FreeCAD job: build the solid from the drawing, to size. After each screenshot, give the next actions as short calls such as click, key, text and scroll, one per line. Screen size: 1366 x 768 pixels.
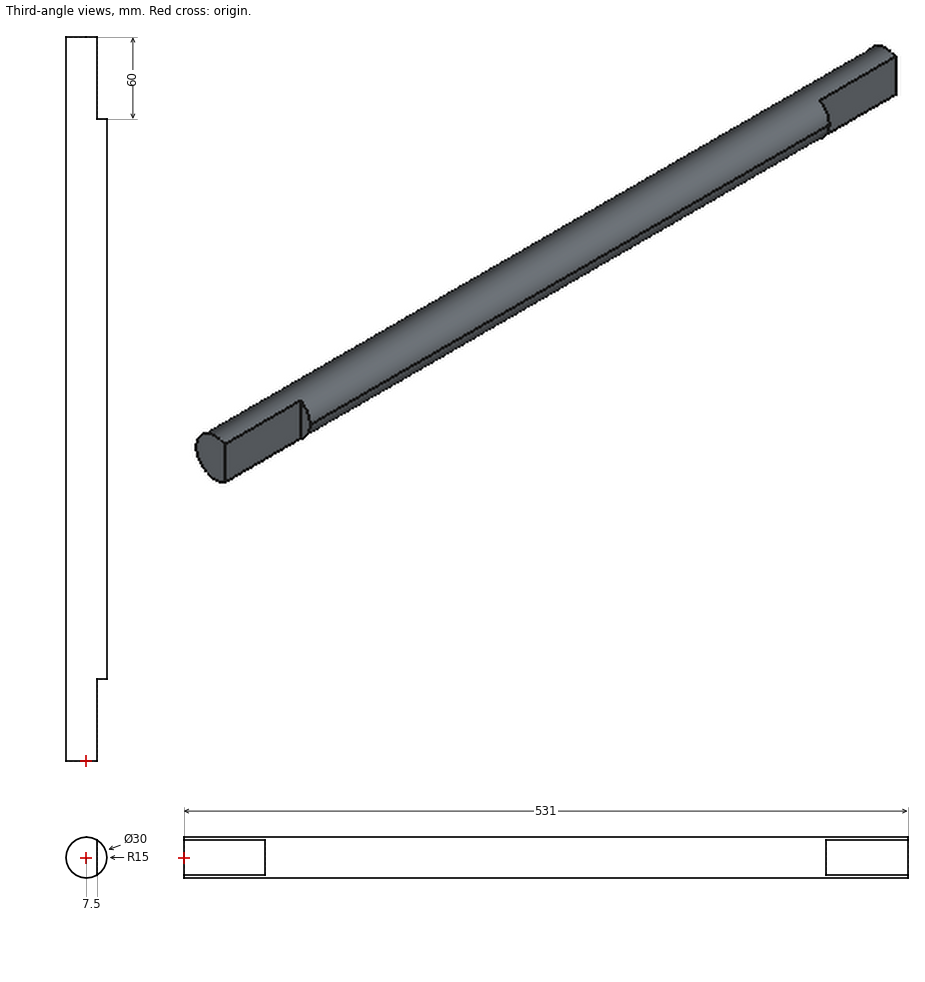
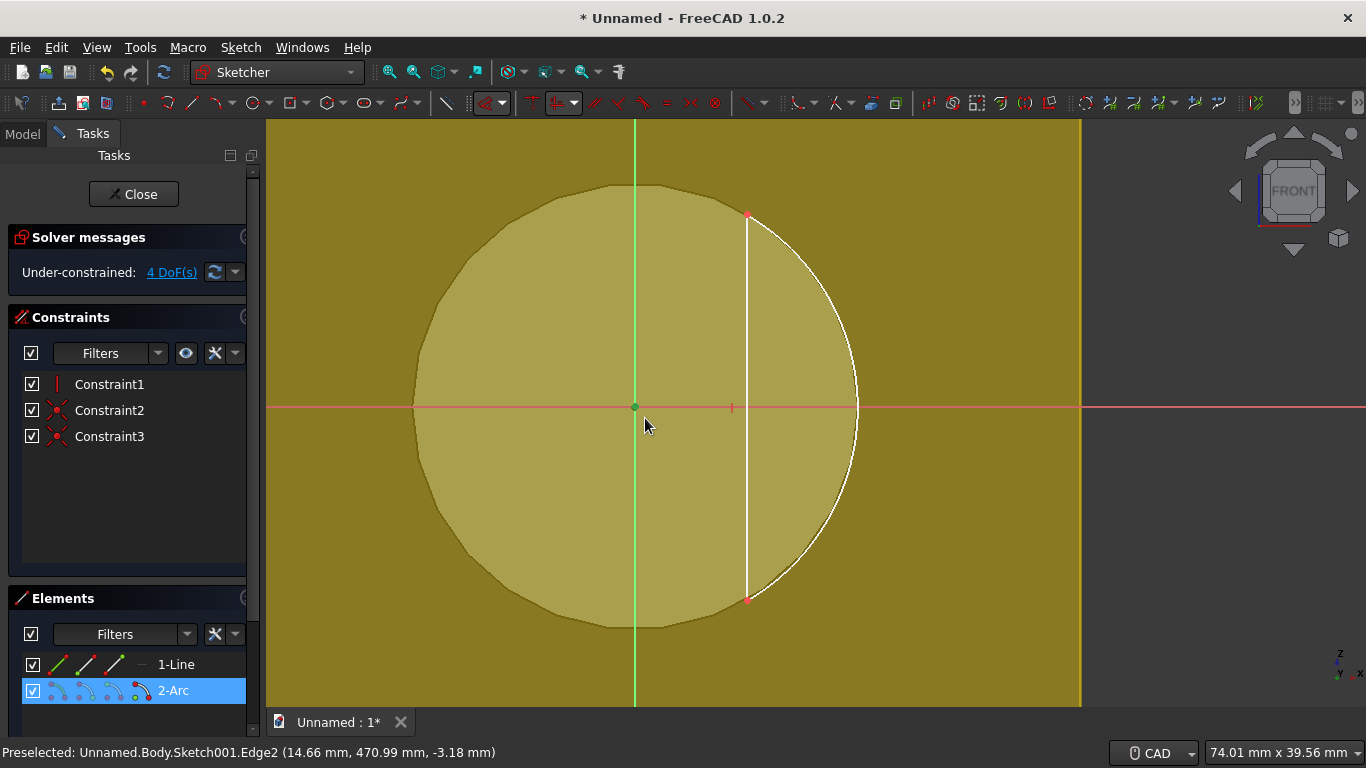
click(532, 104)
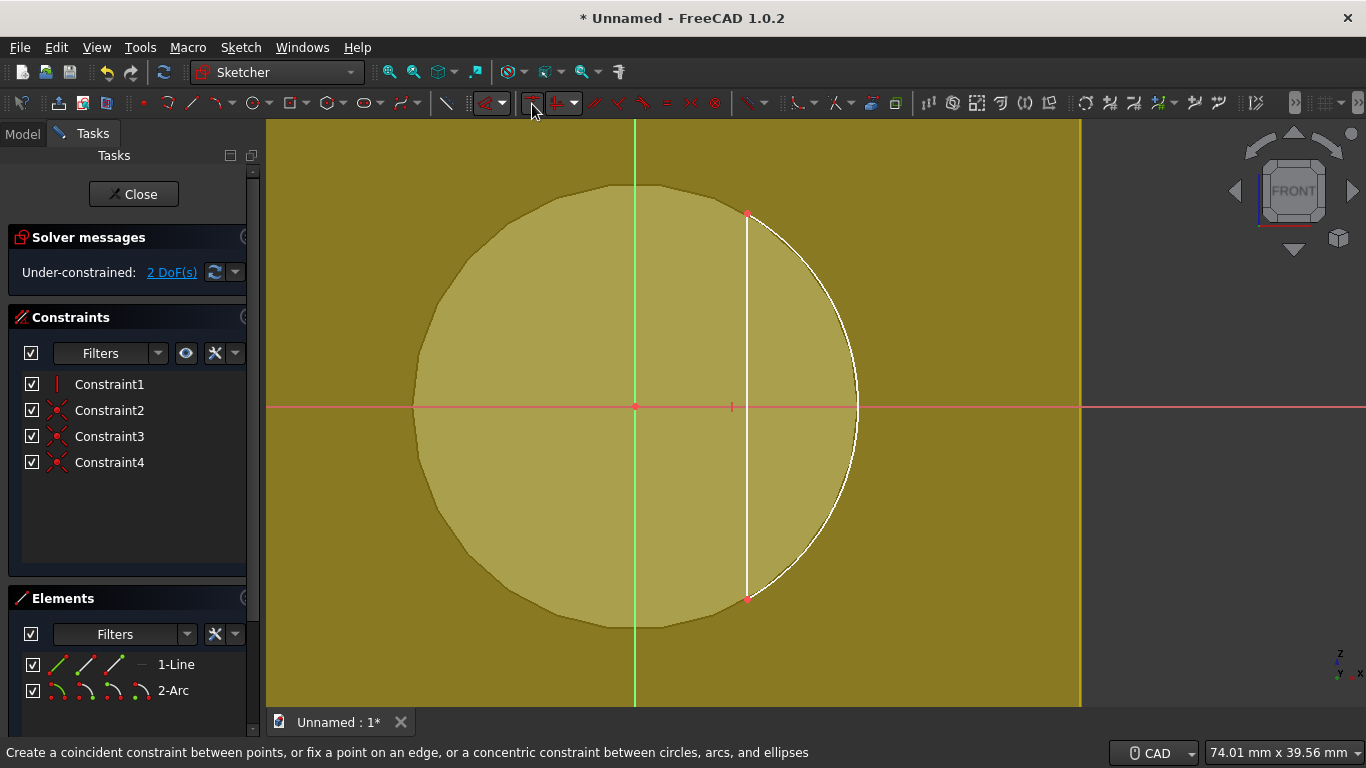
click(486, 104)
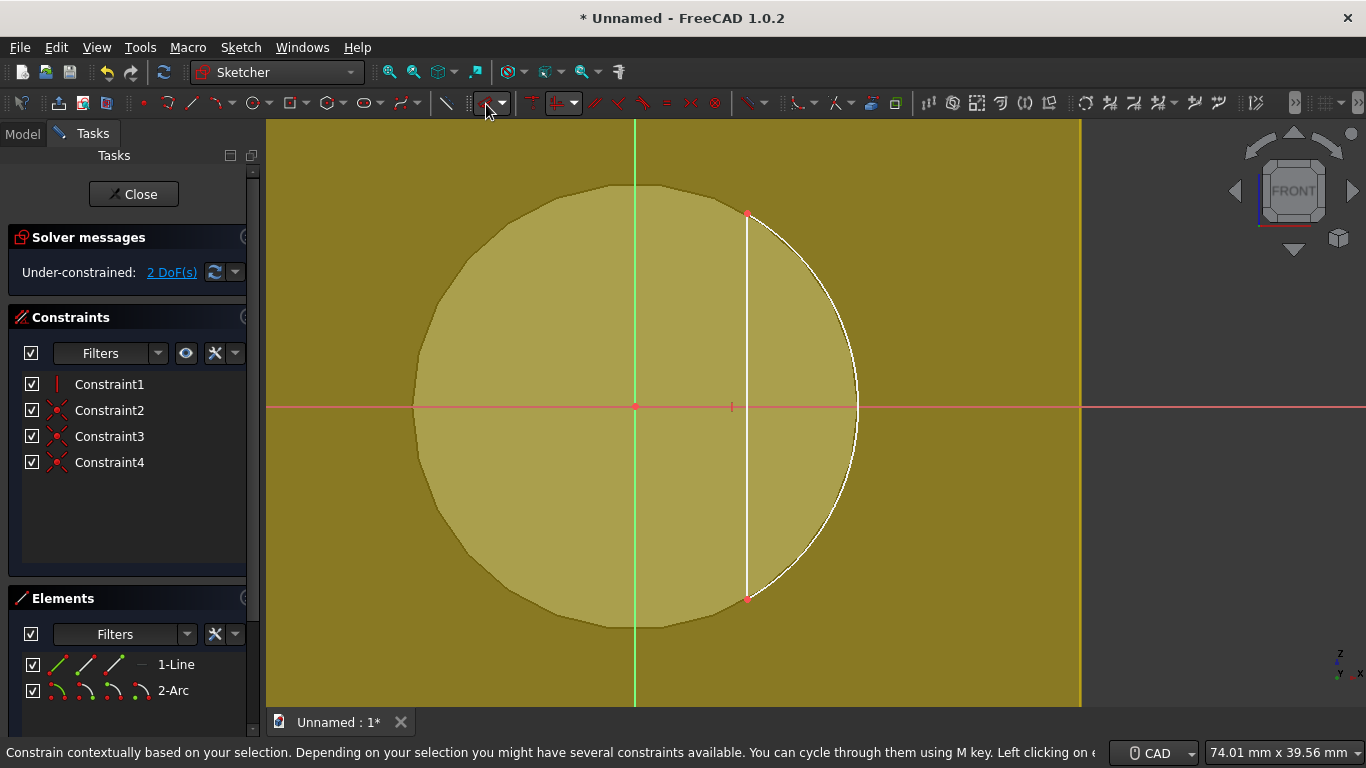
click(839, 497)
click(868, 510)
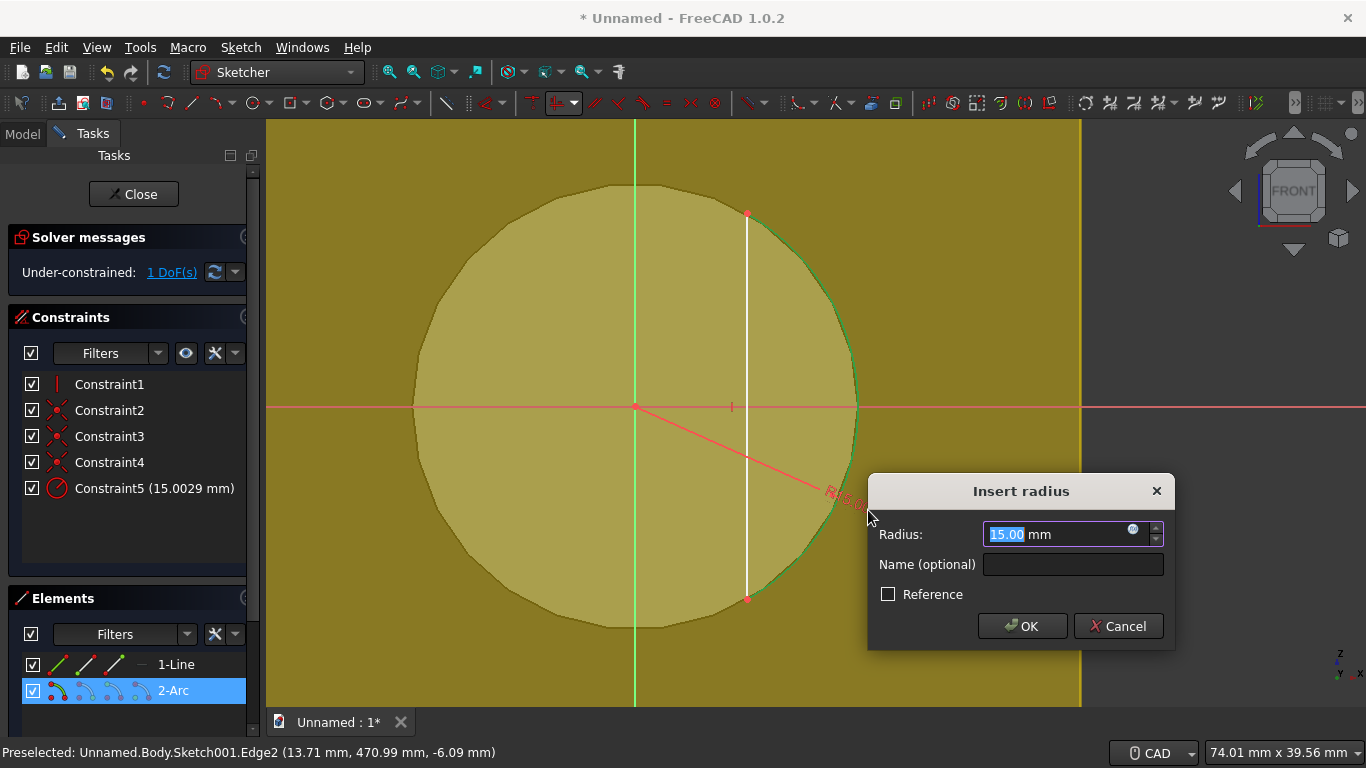
text(15)
key(Return)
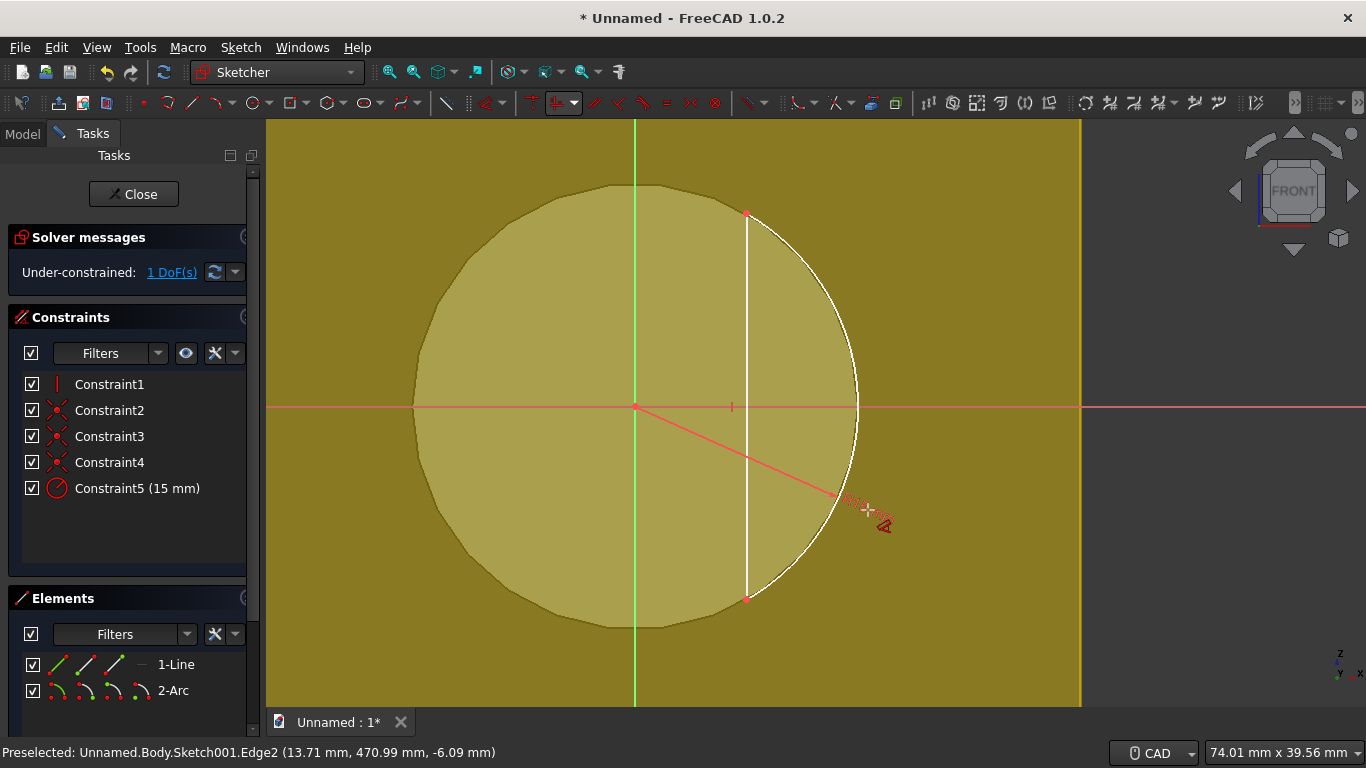
click(747, 600)
click(691, 634)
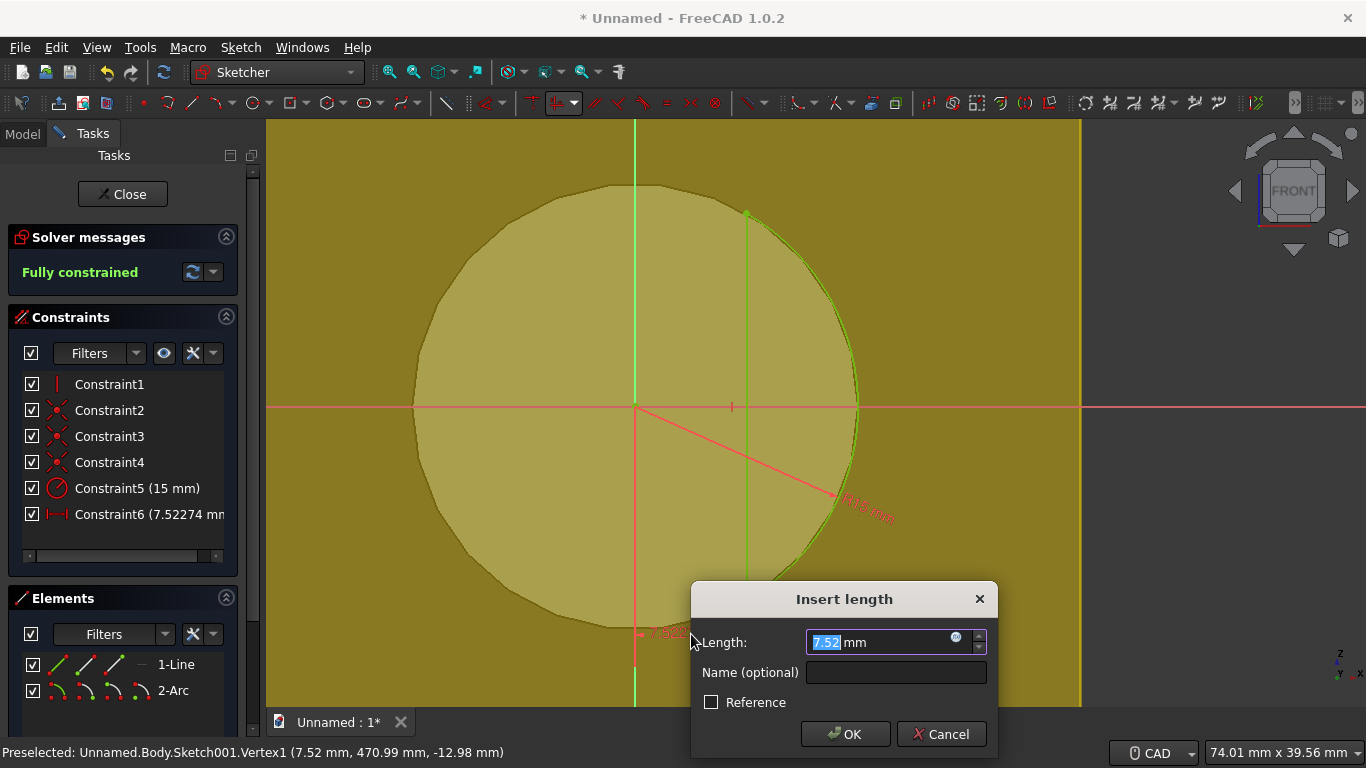
text(7.5)
key(Return)
key(Escape)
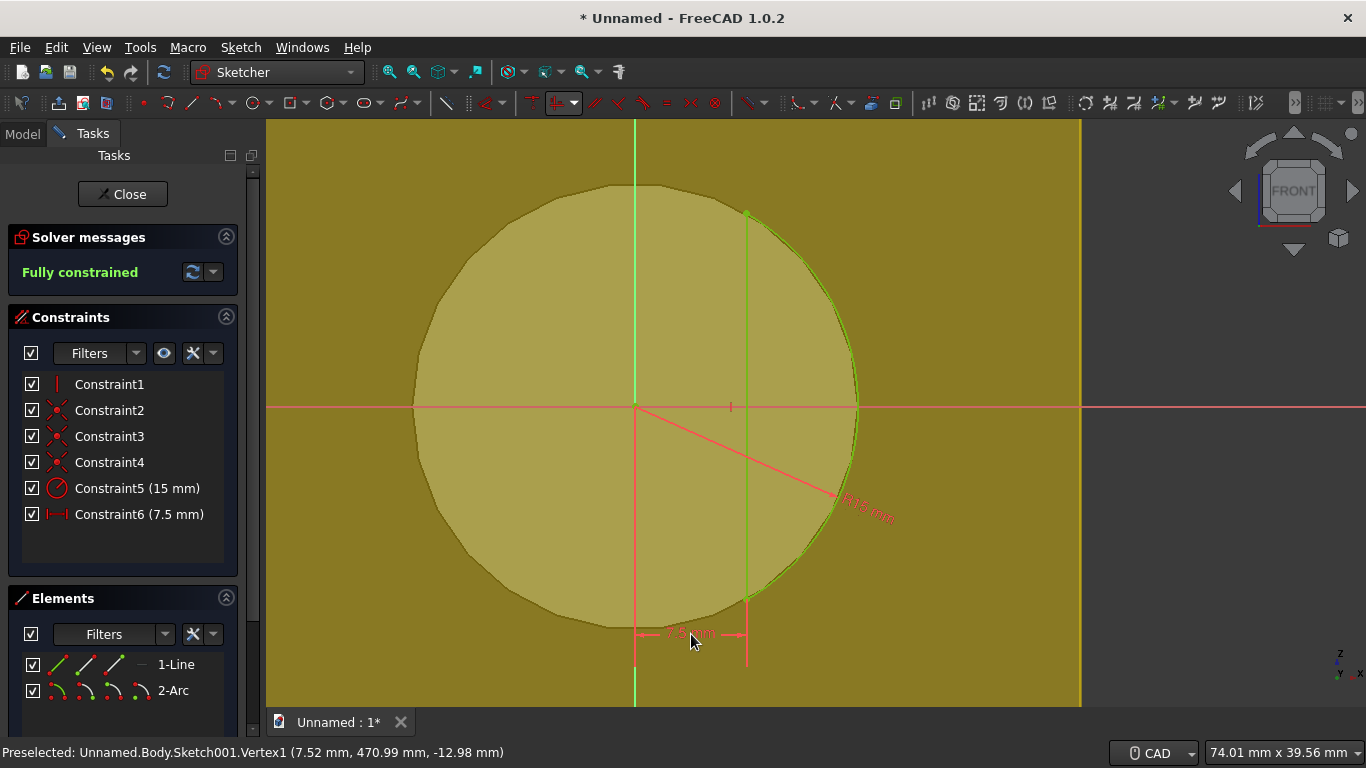
click(123, 194)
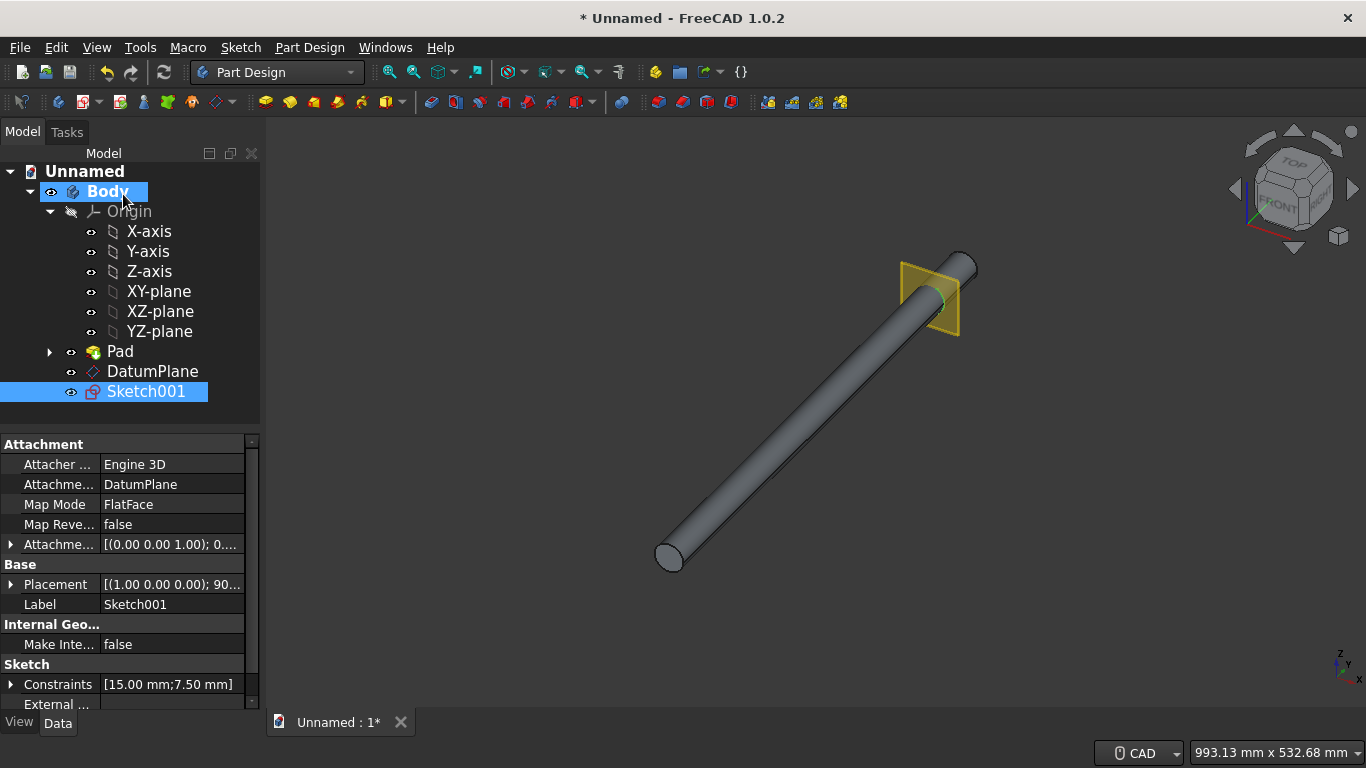
click(432, 102)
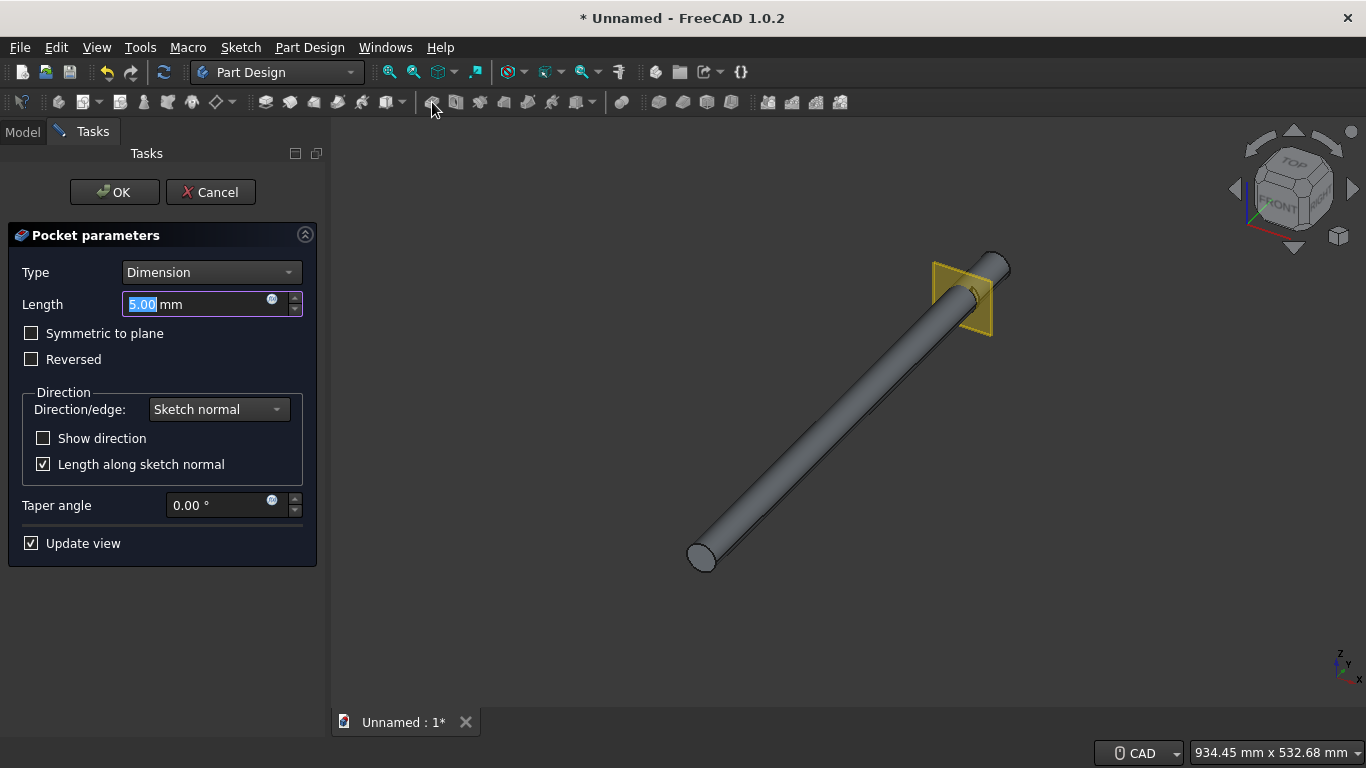
text(60)
key(Tab)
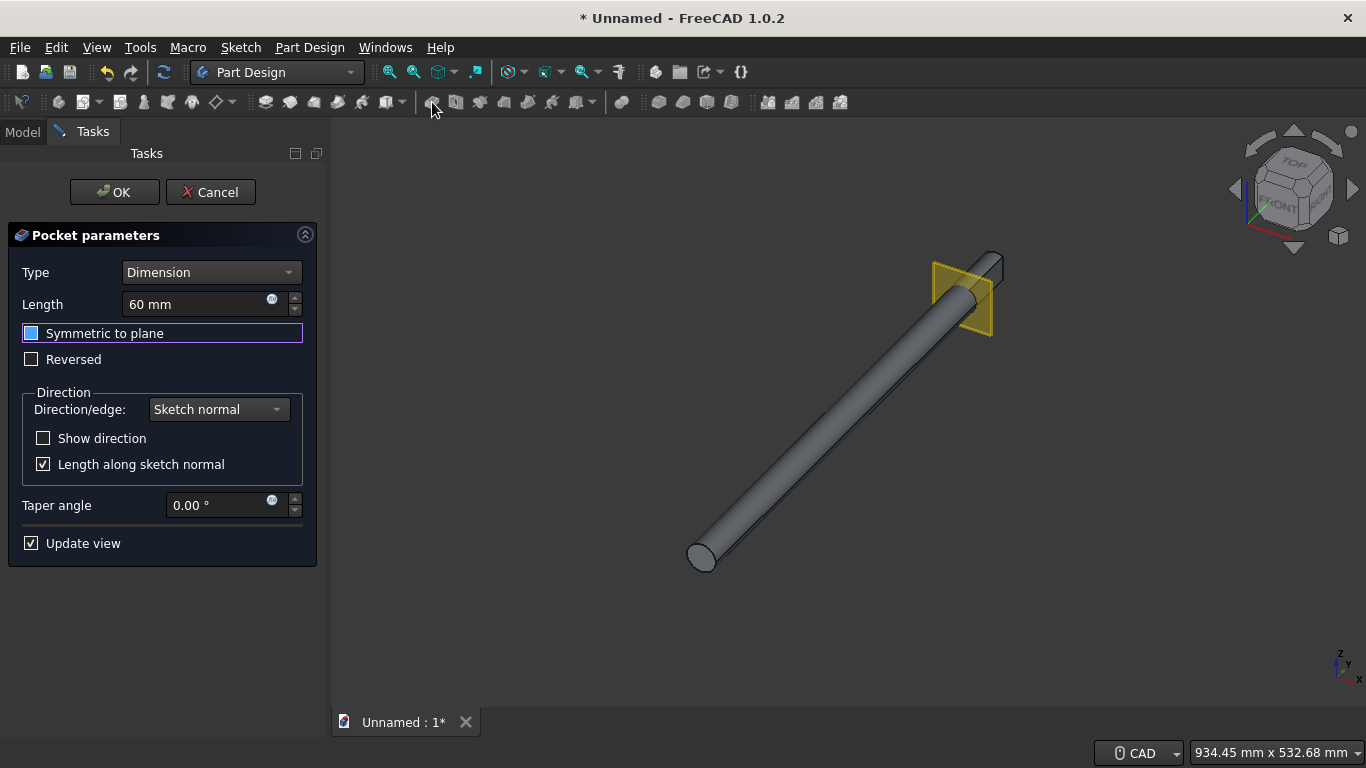
click(115, 192)